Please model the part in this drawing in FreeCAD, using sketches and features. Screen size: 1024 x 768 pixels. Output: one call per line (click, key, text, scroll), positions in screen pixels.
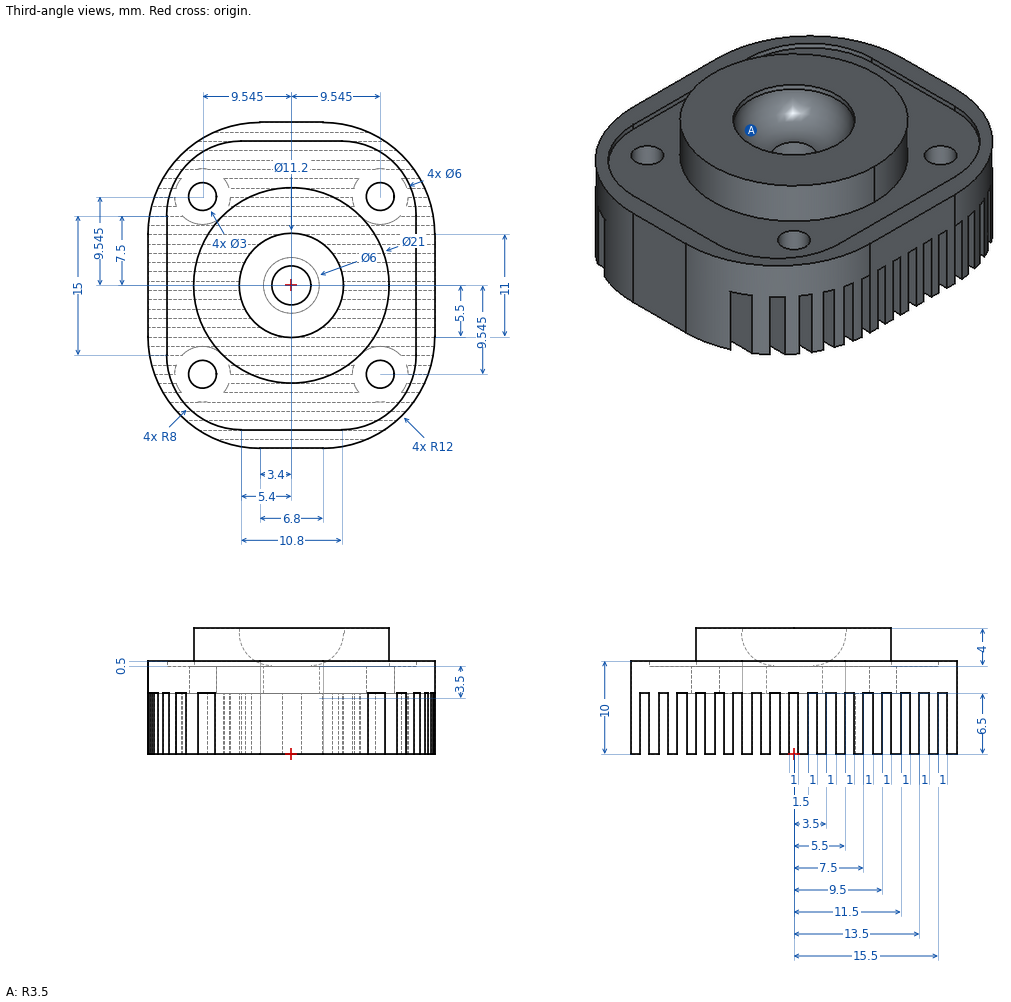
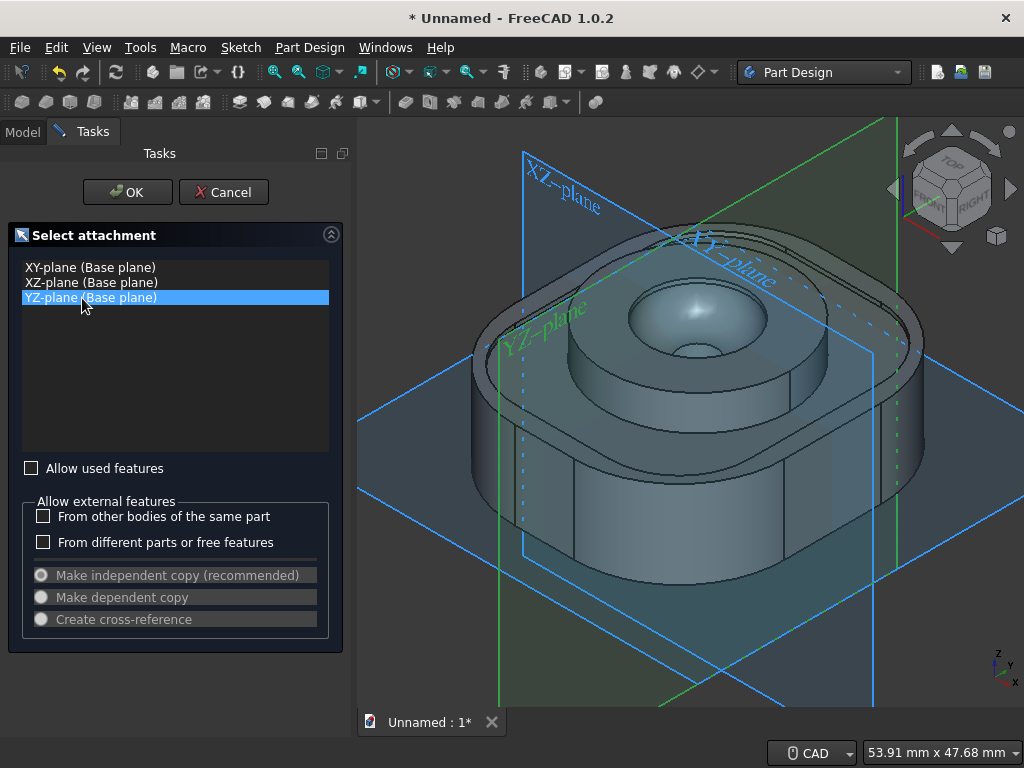
click(128, 192)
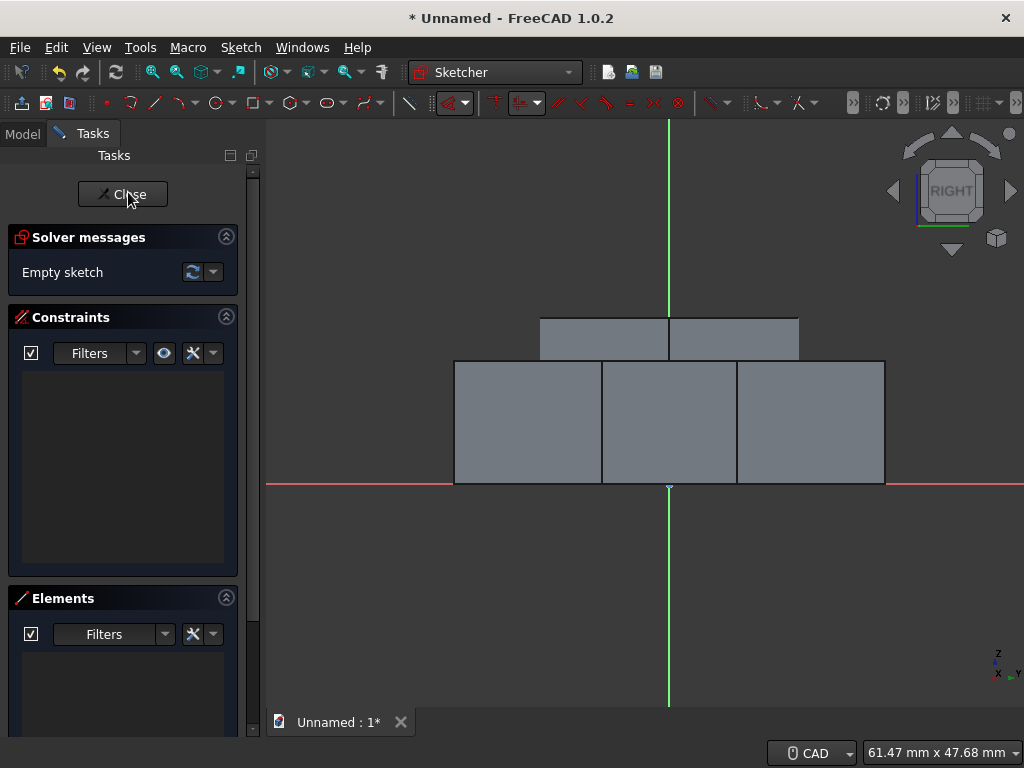
click(70, 104)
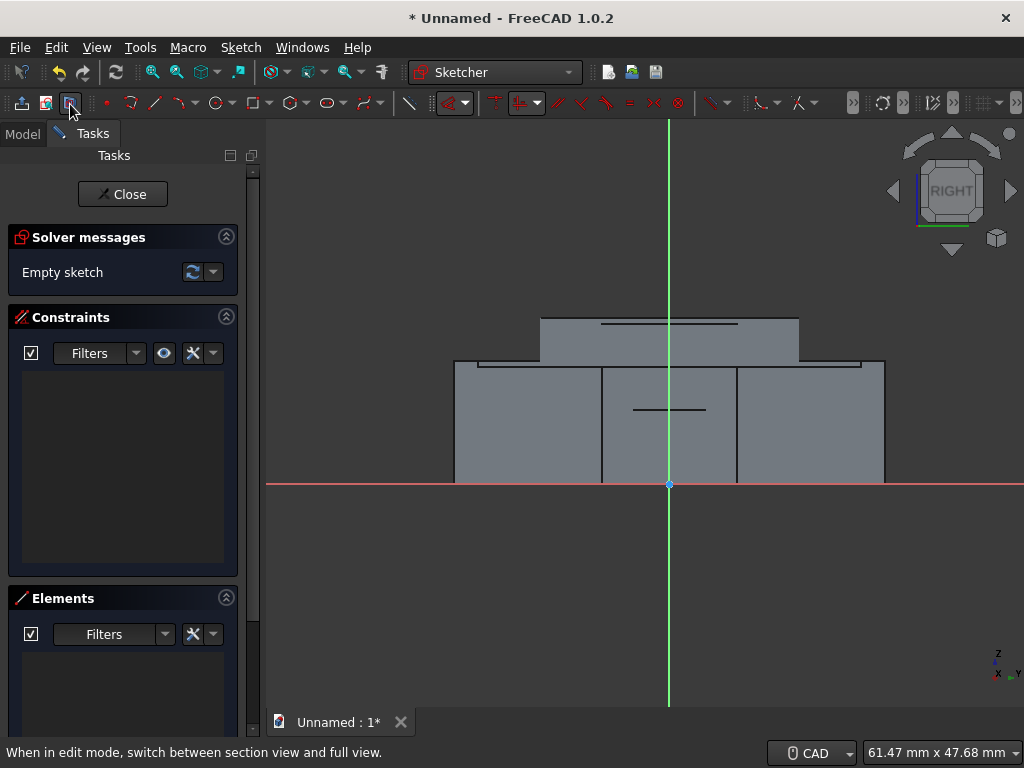
scroll(576, 413, down, 5)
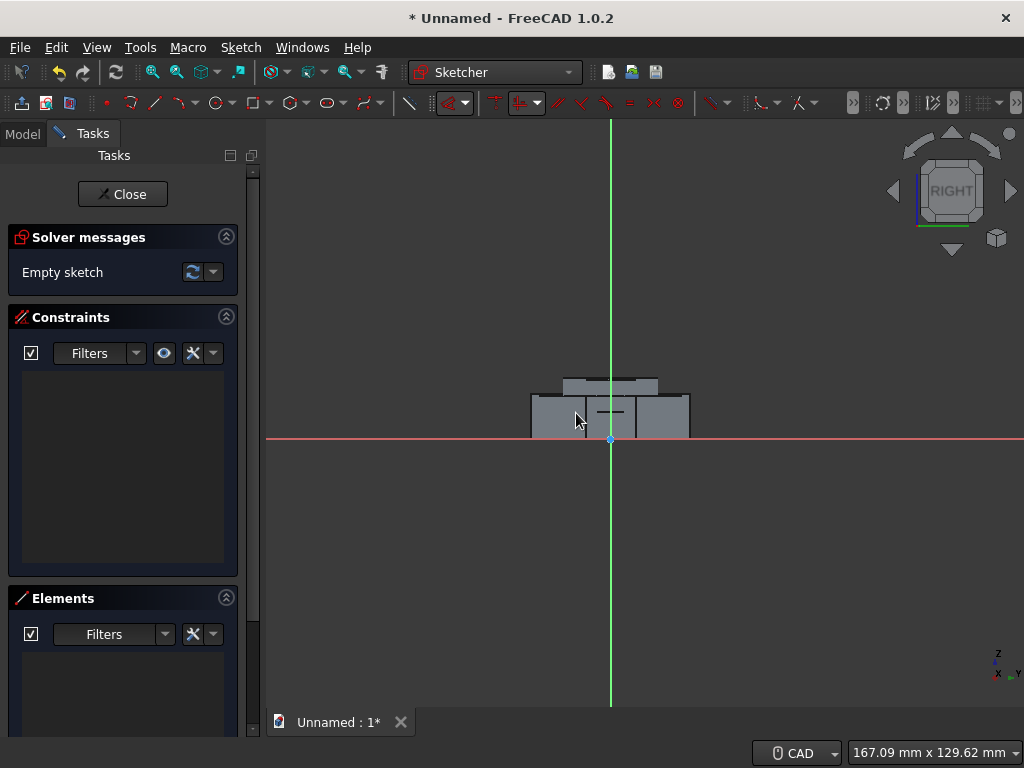
scroll(665, 428, up, 8)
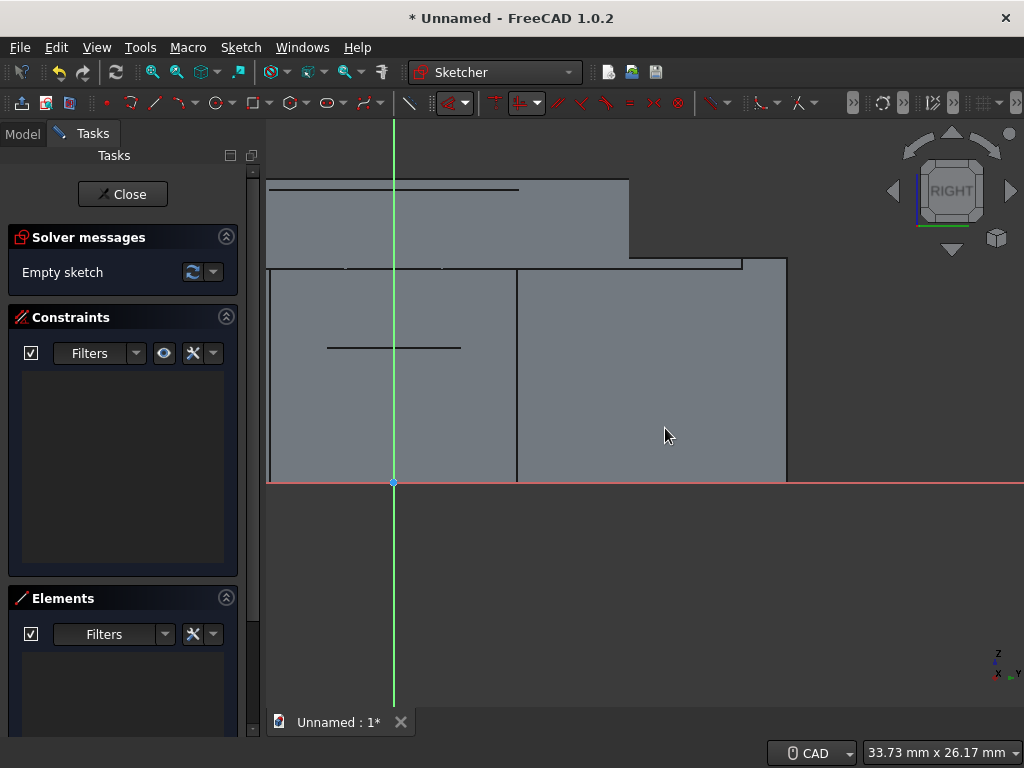
click(254, 104)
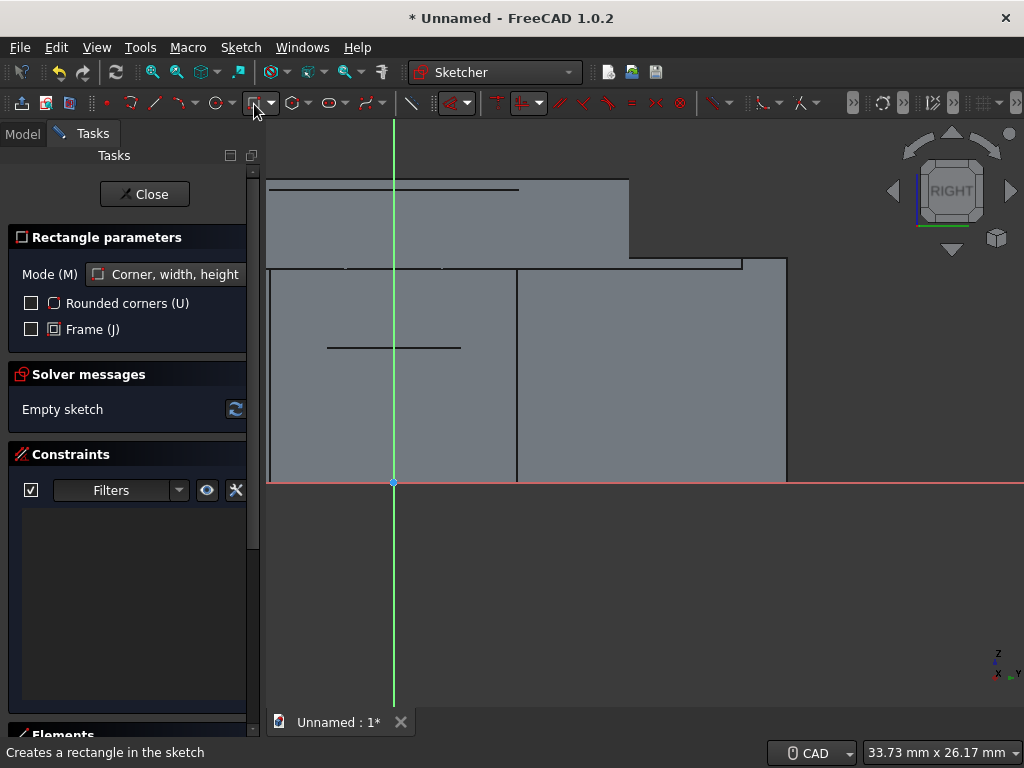
click(427, 337)
click(450, 483)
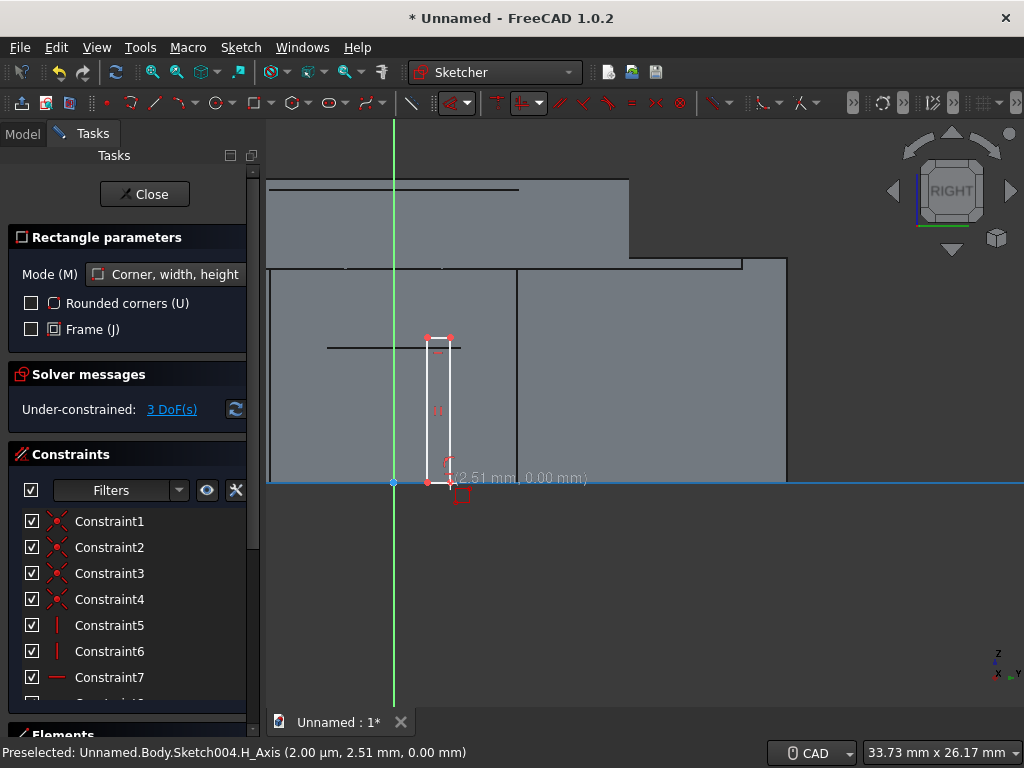
scroll(382, 337, up, 2)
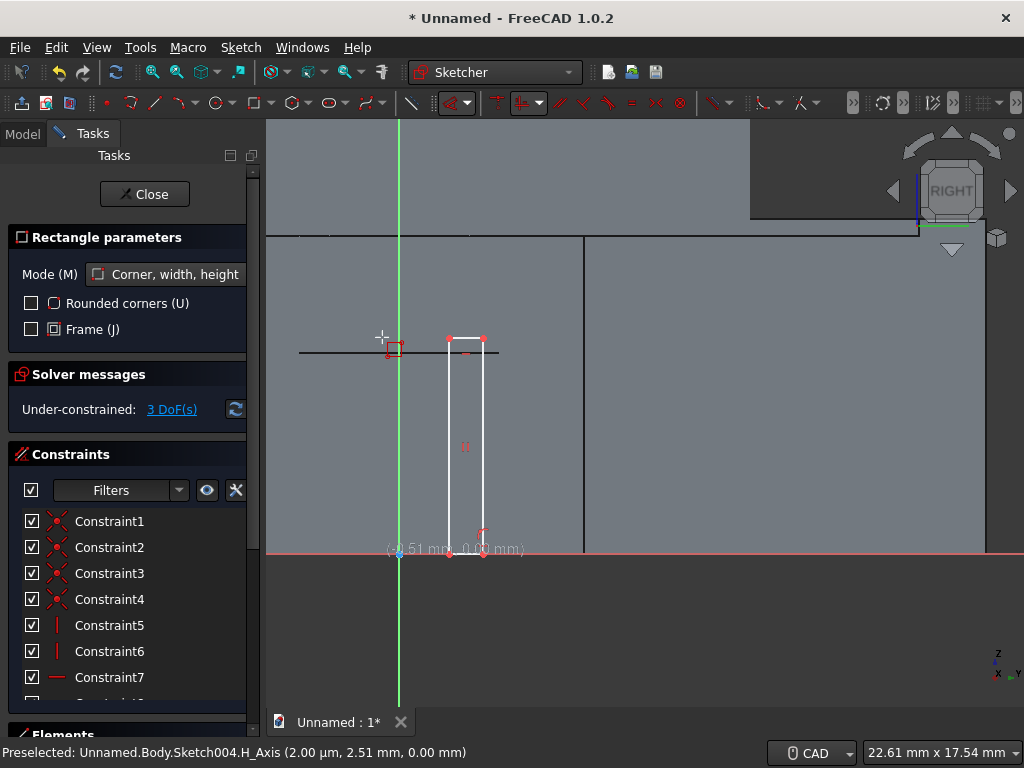
click(382, 336)
click(416, 554)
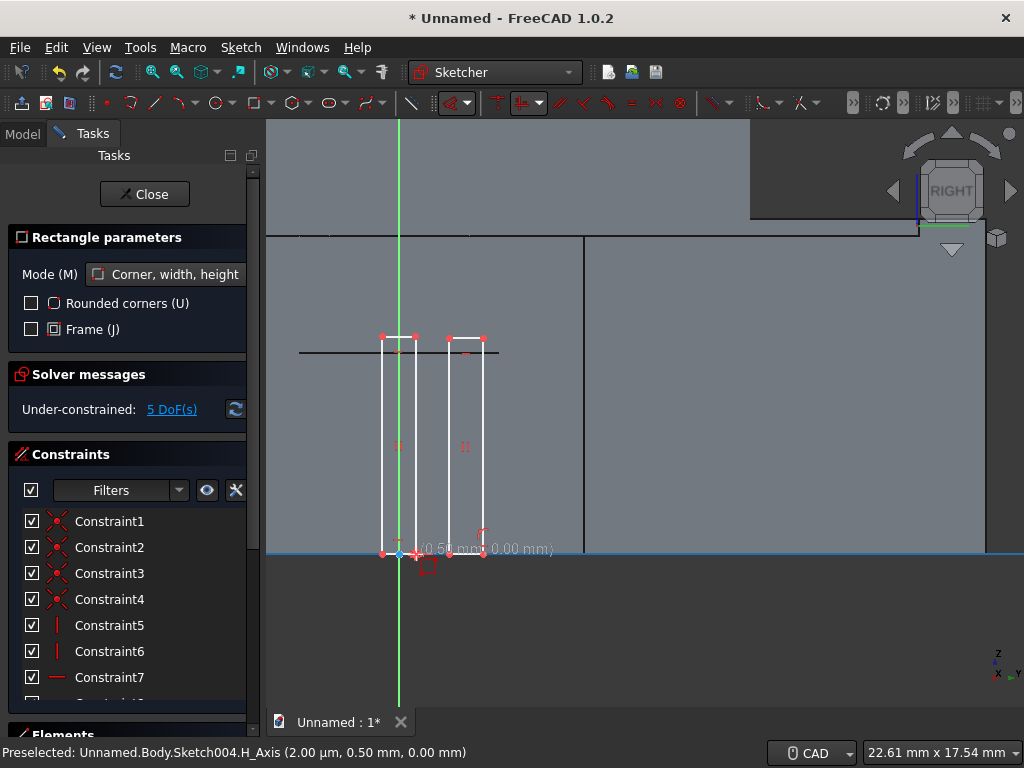
click(516, 336)
click(550, 554)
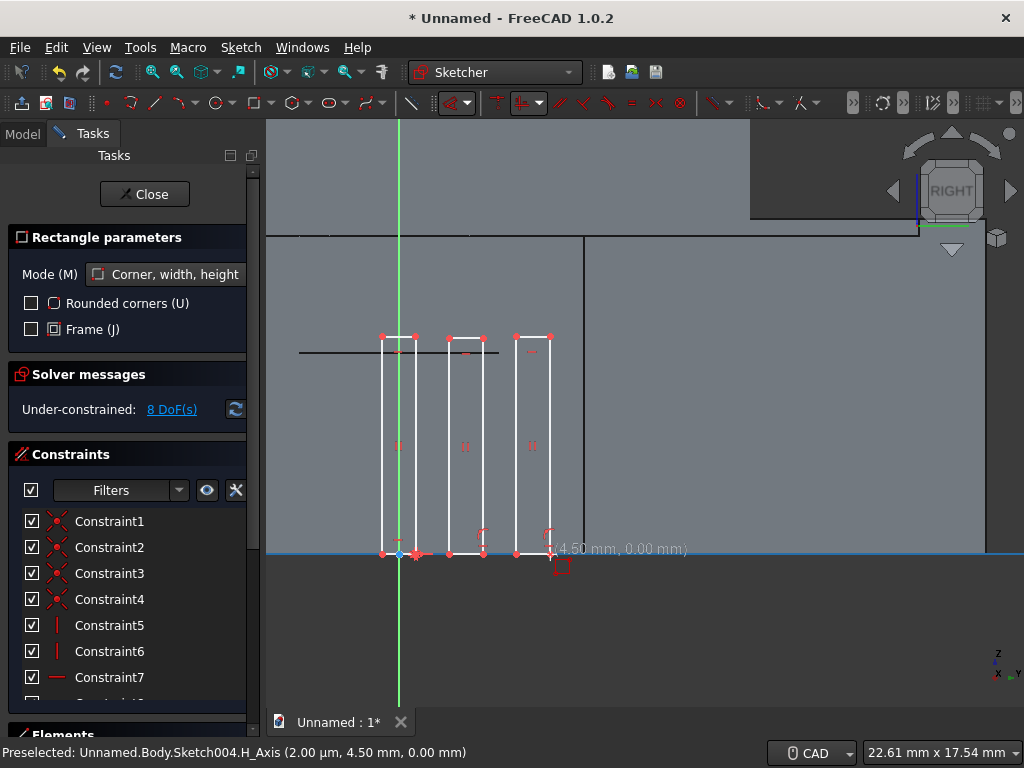
click(584, 336)
click(617, 554)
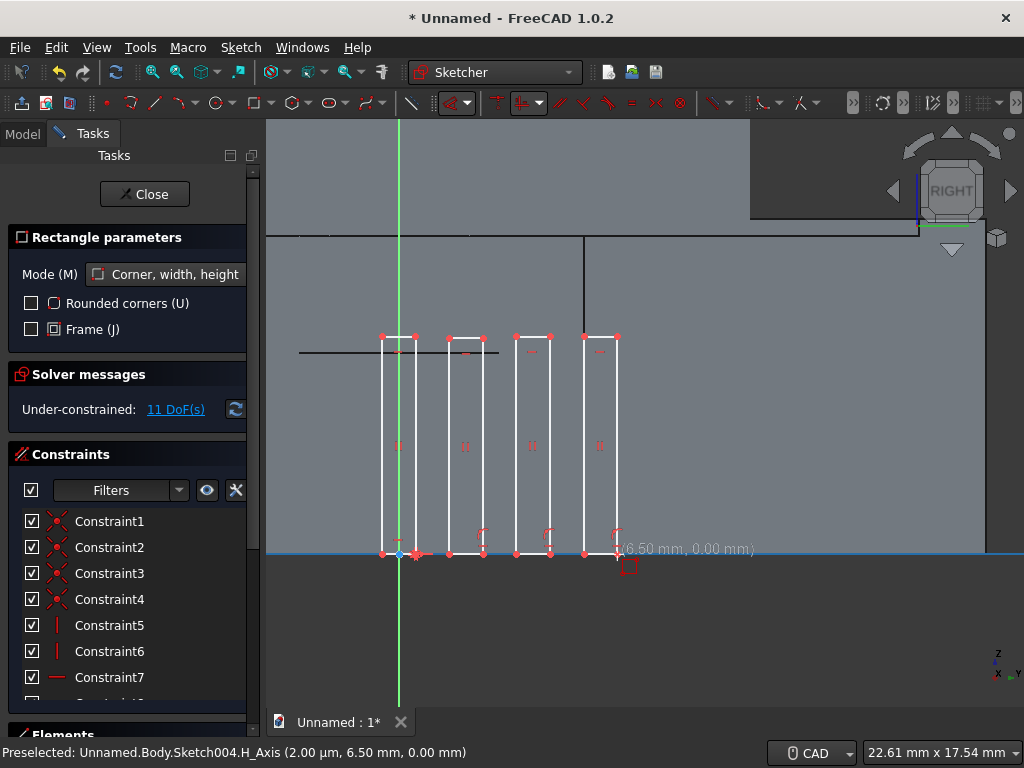
click(651, 336)
click(684, 554)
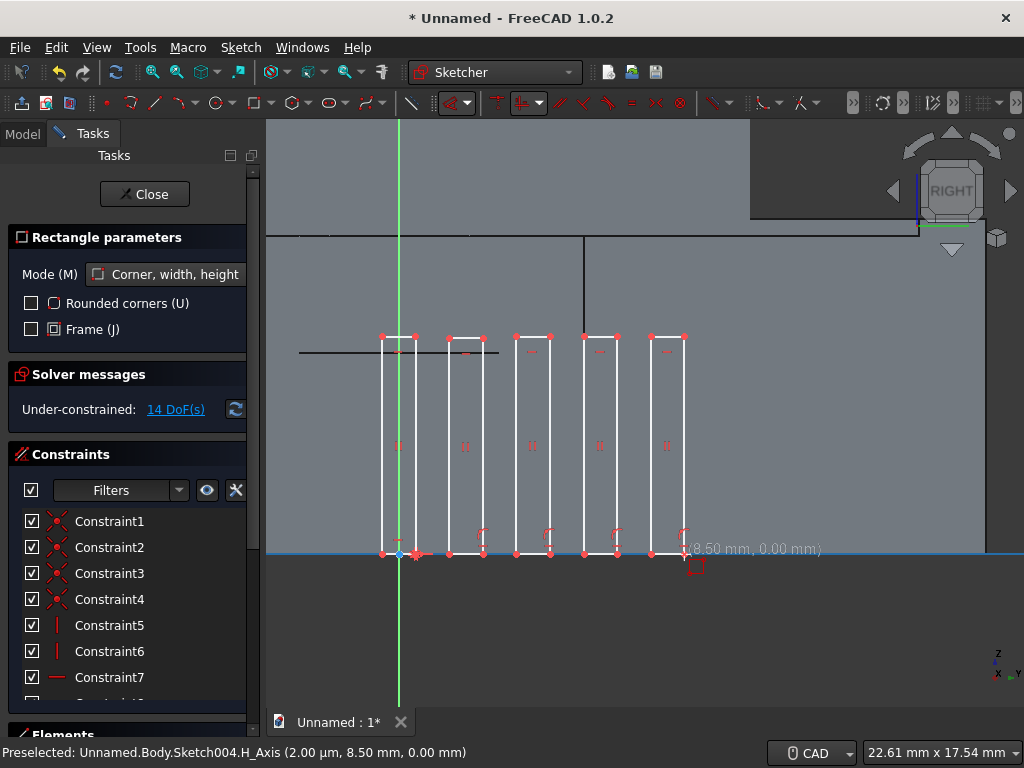
click(718, 336)
click(751, 554)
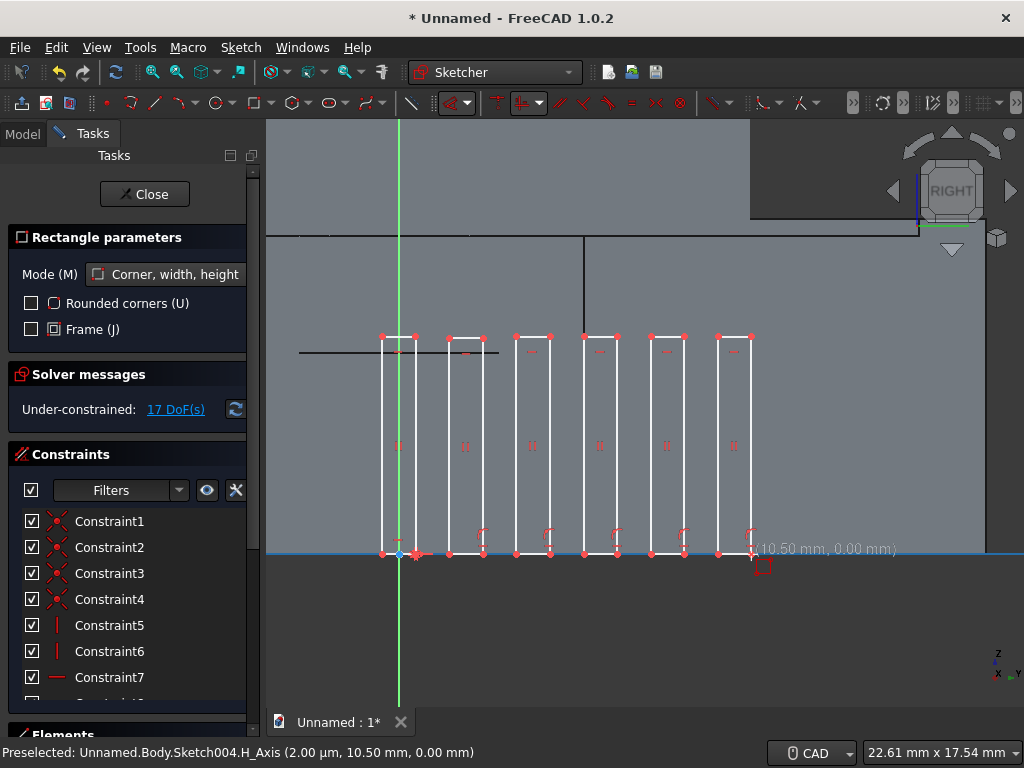
click(785, 336)
click(818, 554)